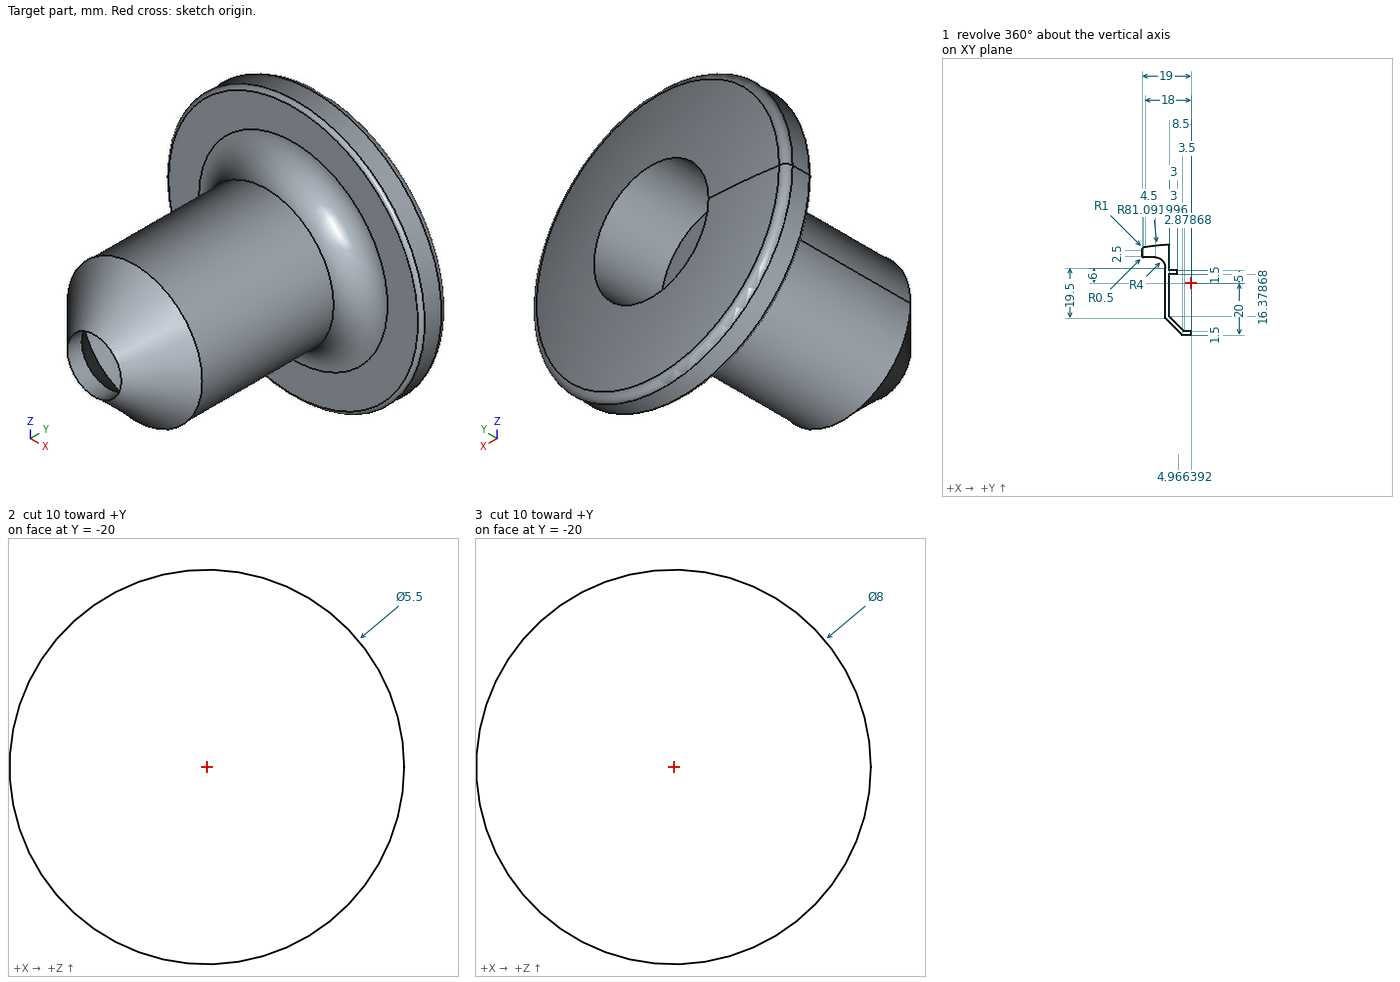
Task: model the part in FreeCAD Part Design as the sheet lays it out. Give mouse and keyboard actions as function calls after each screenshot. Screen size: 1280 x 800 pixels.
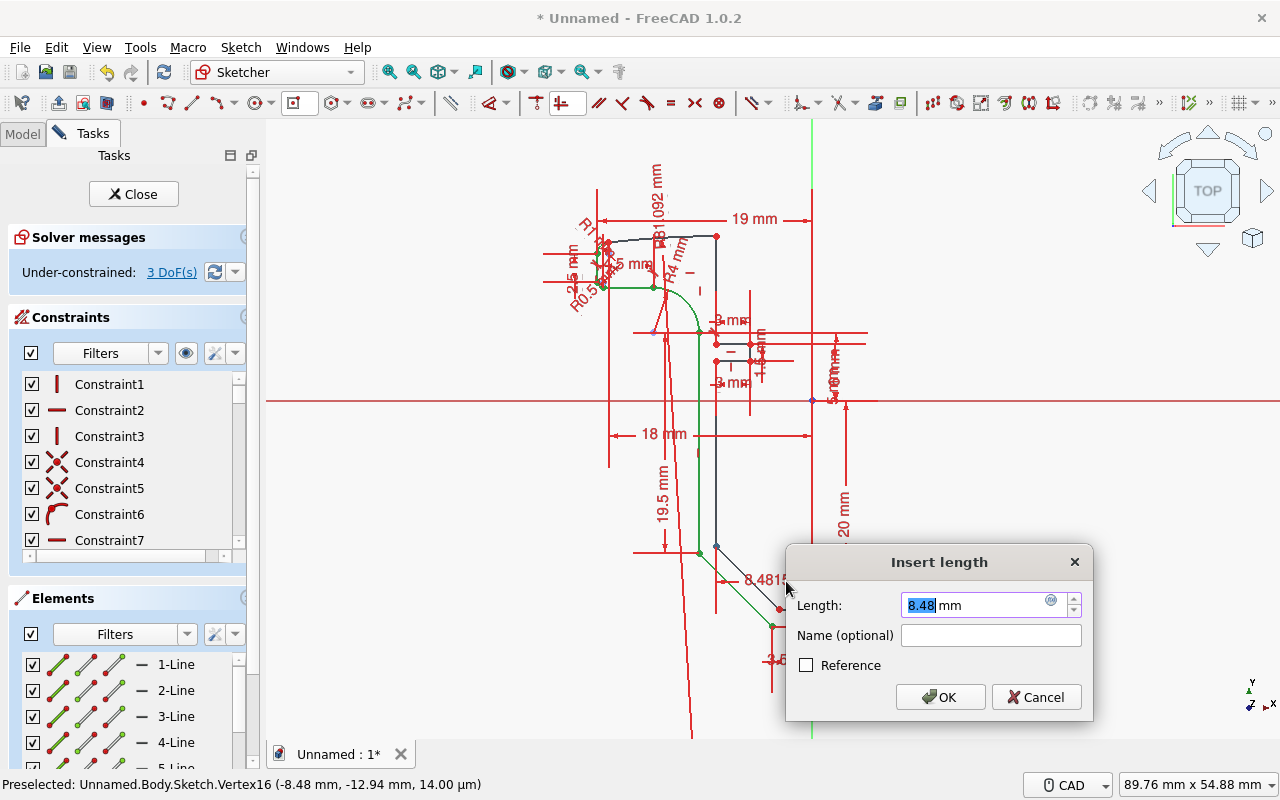
text(8.5)
key(Return)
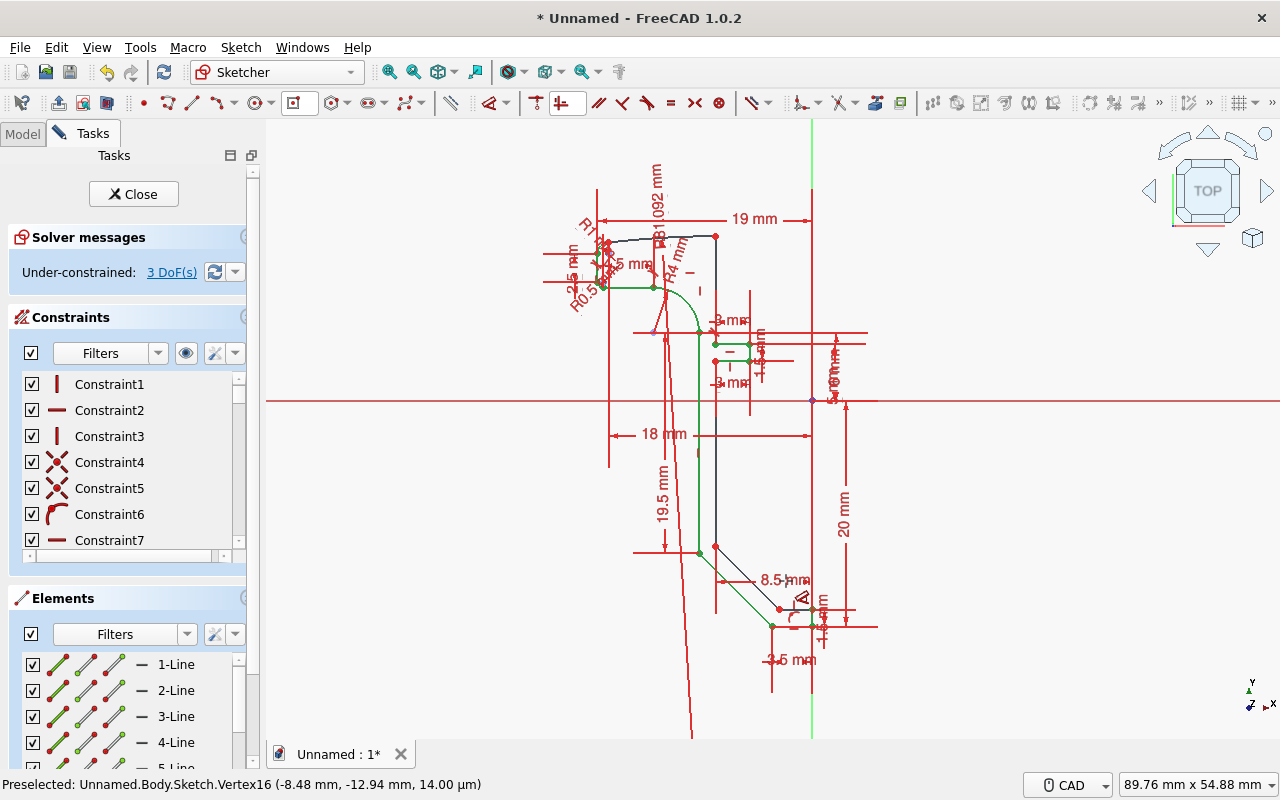
scroll(802, 610, up, 2)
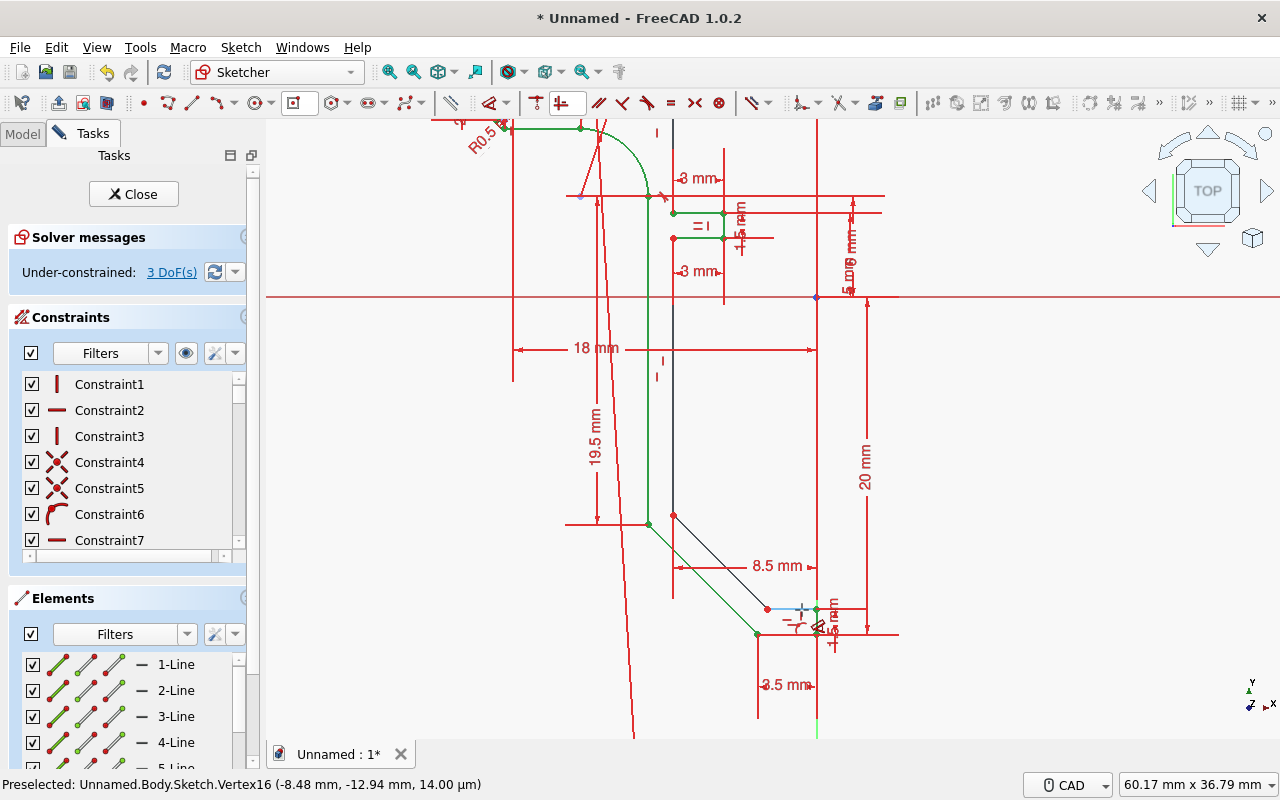
click(802, 609)
click(792, 527)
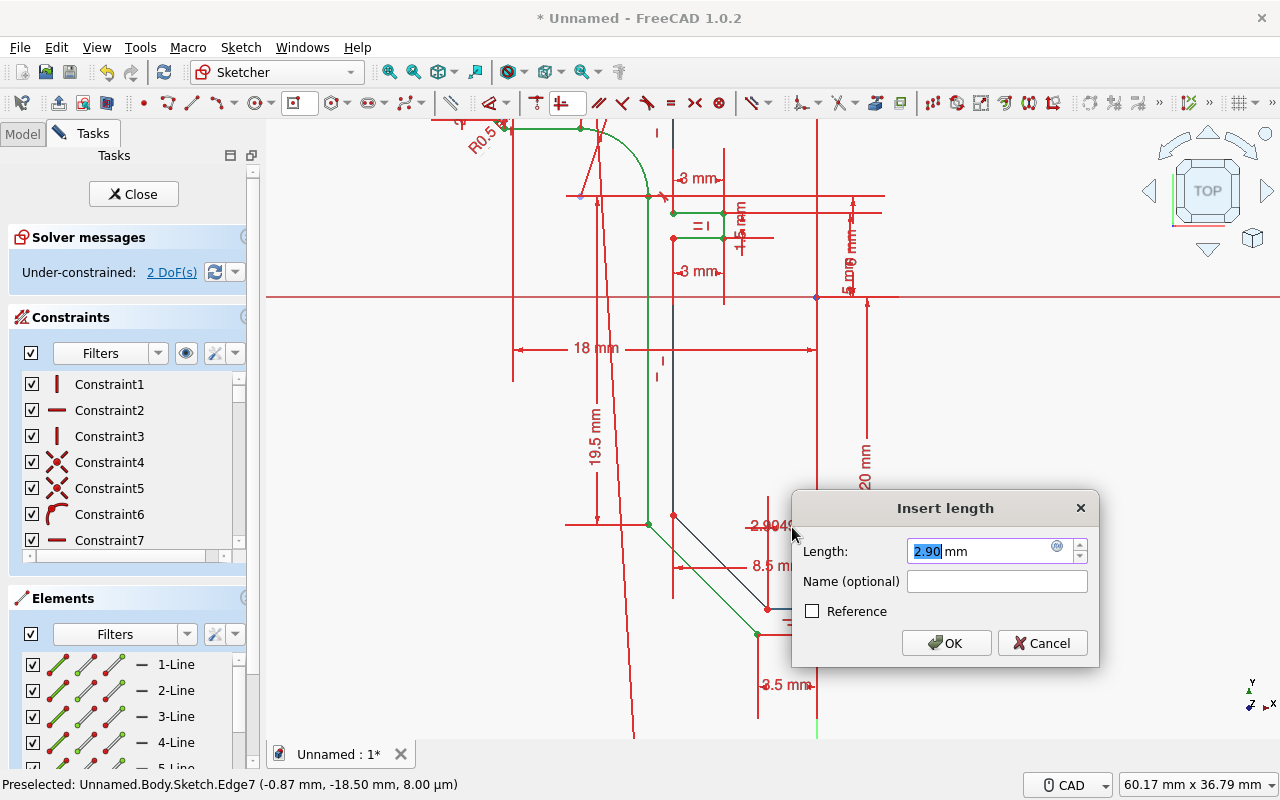
text(2.87868)
key(Return)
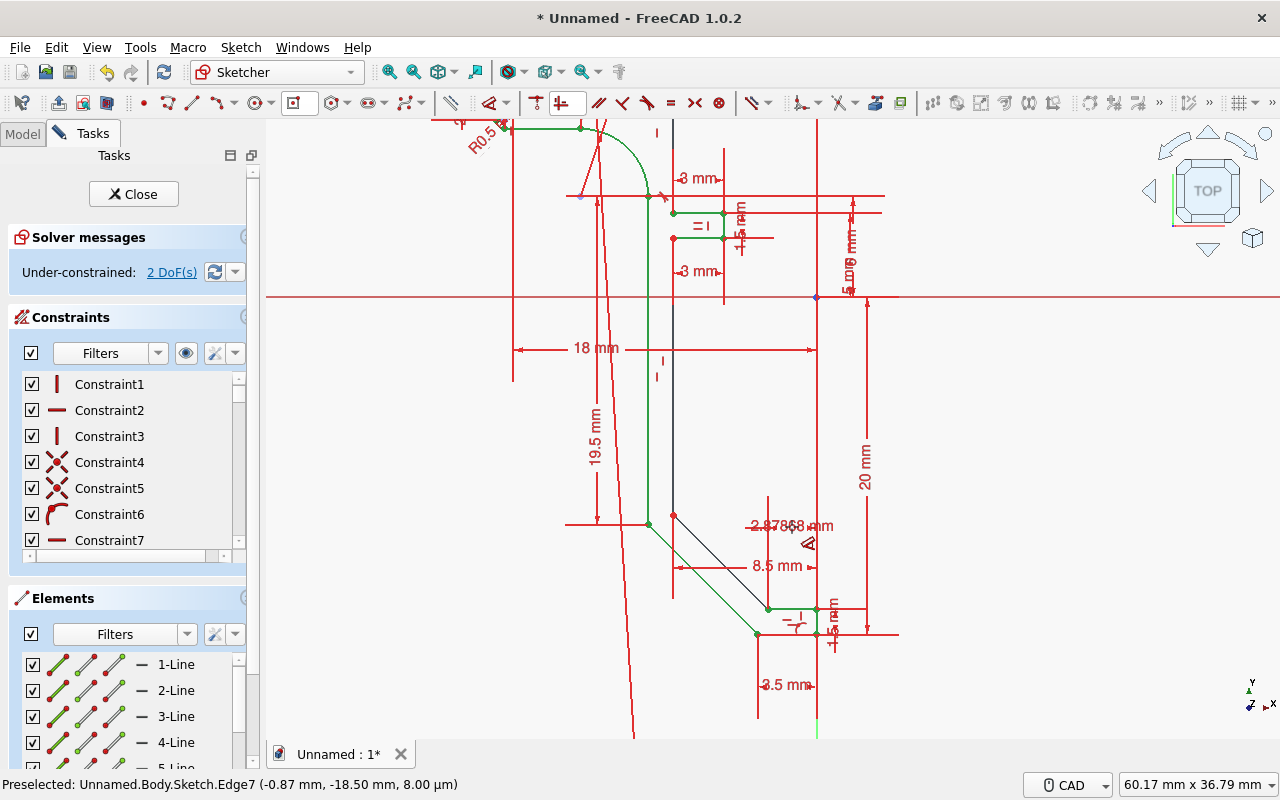
click(673, 432)
click(707, 377)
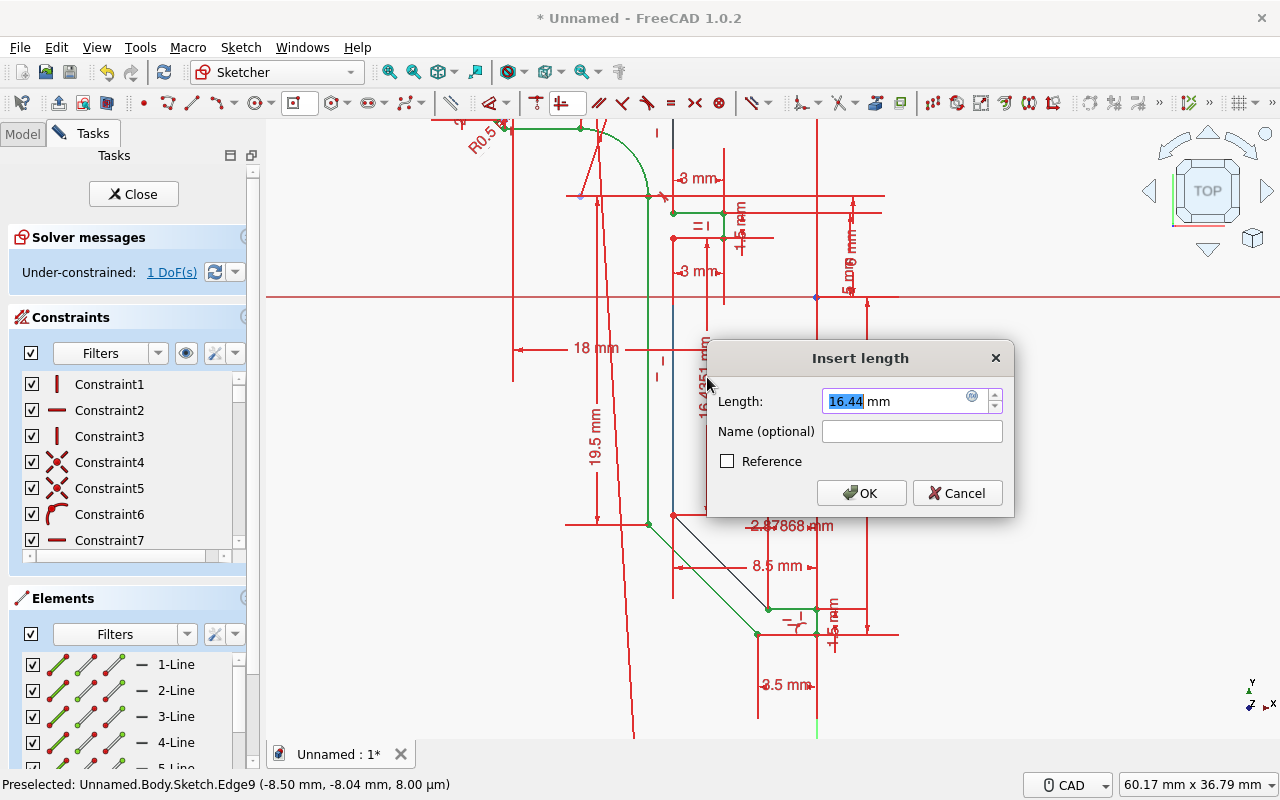
text(16.37868)
key(Return)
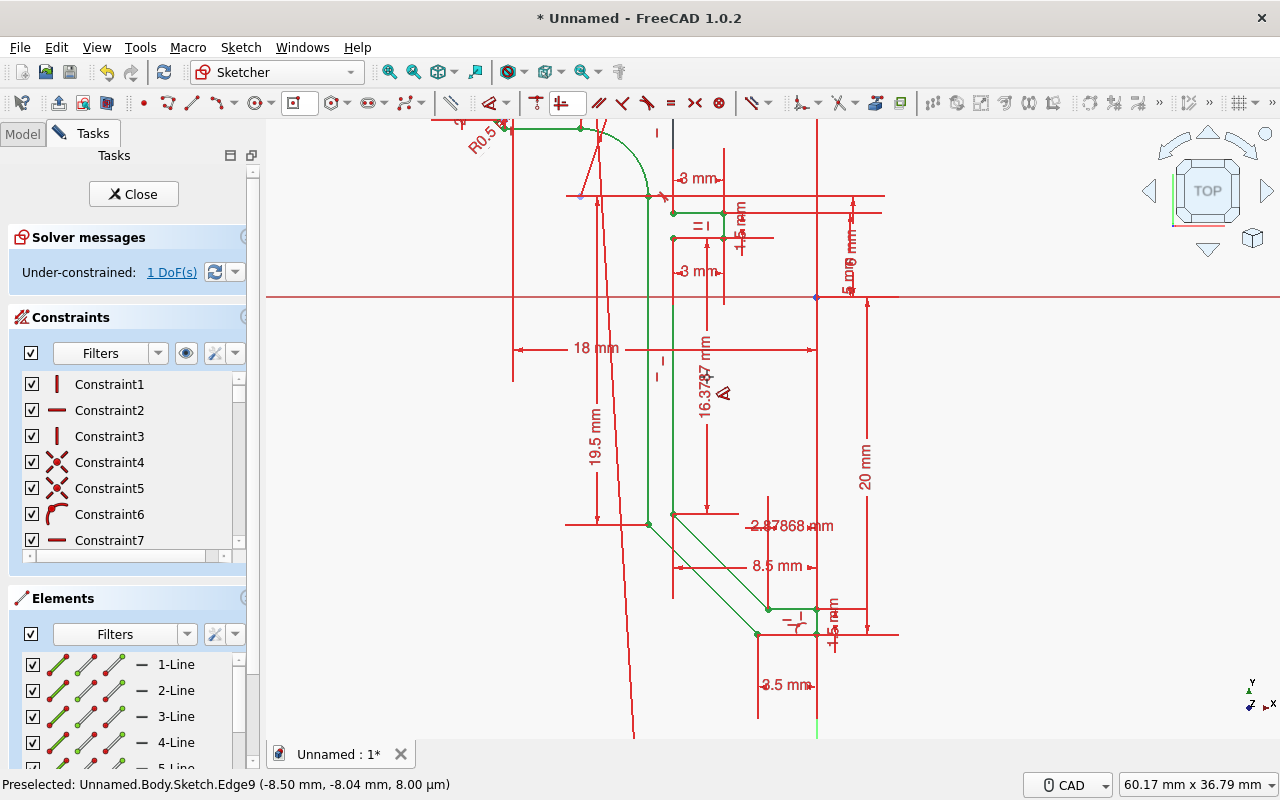
scroll(802, 610, down, 2)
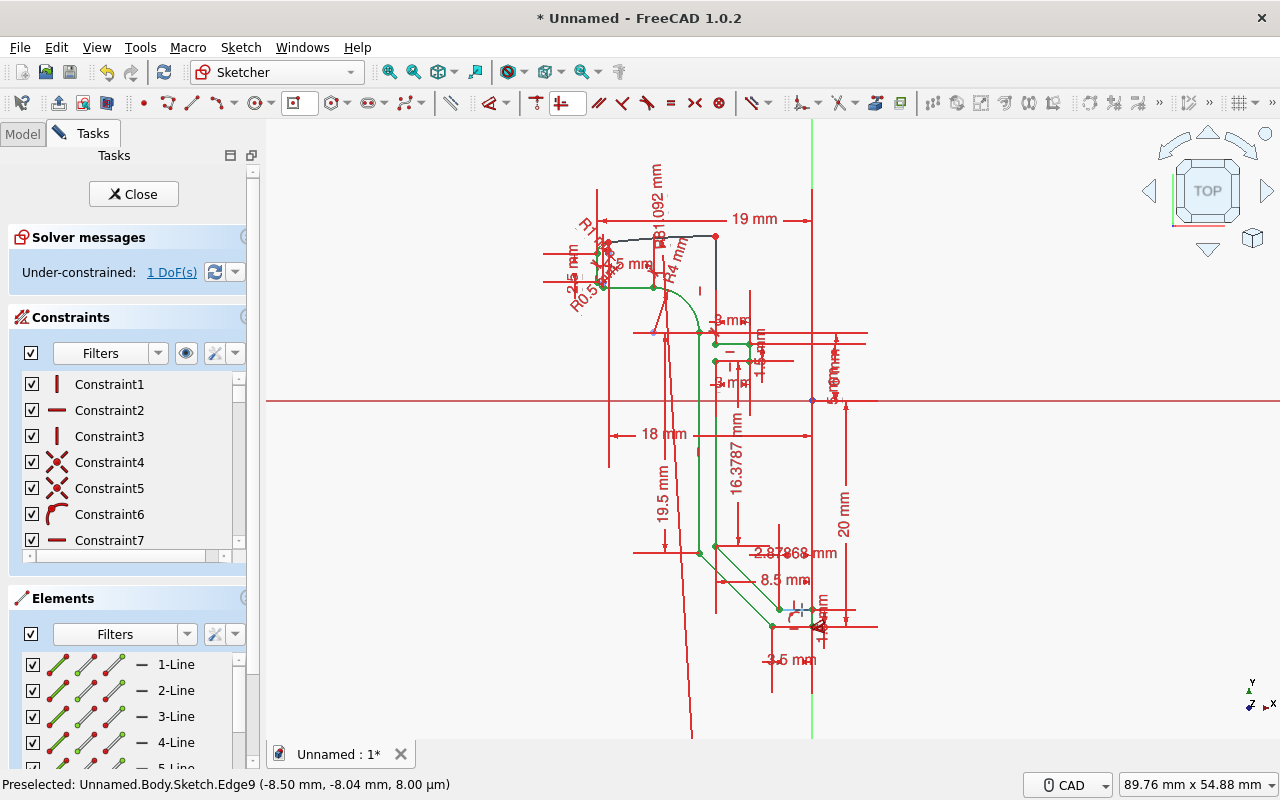
scroll(704, 214, down, 4)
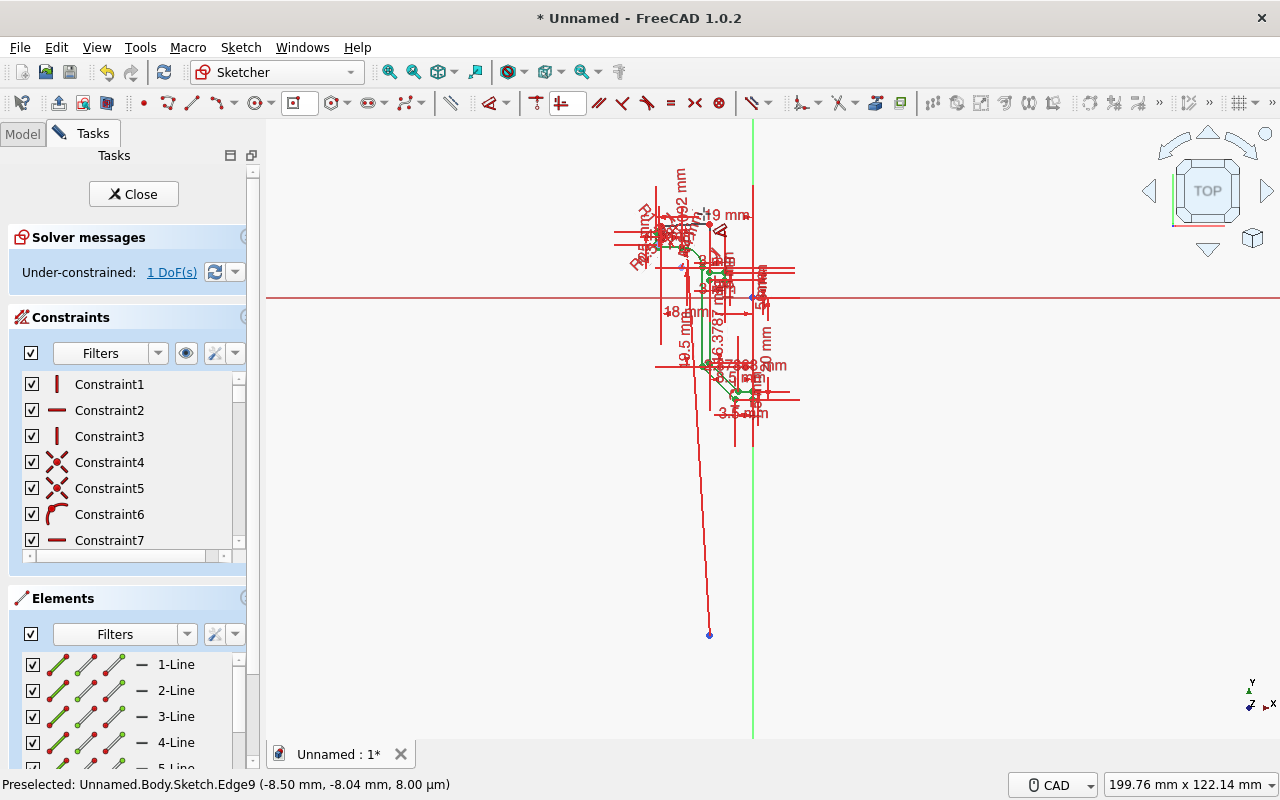
scroll(710, 636, up, 3)